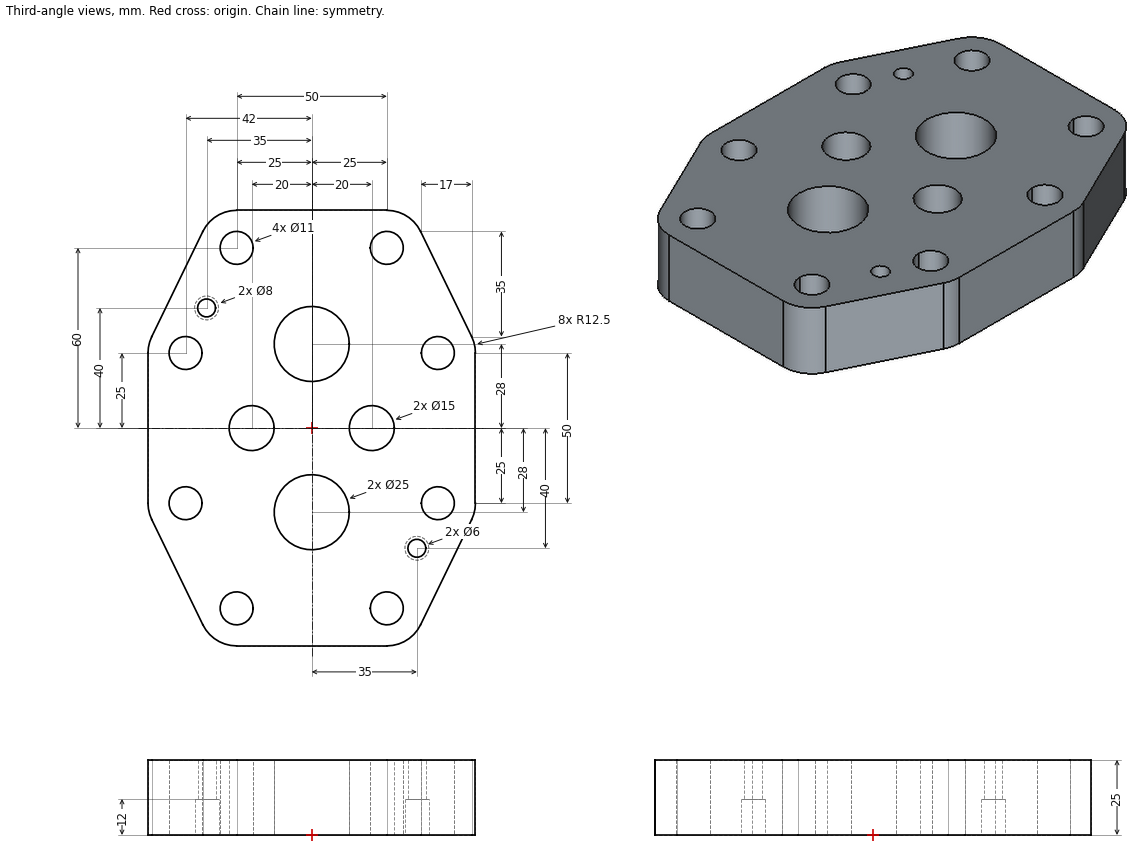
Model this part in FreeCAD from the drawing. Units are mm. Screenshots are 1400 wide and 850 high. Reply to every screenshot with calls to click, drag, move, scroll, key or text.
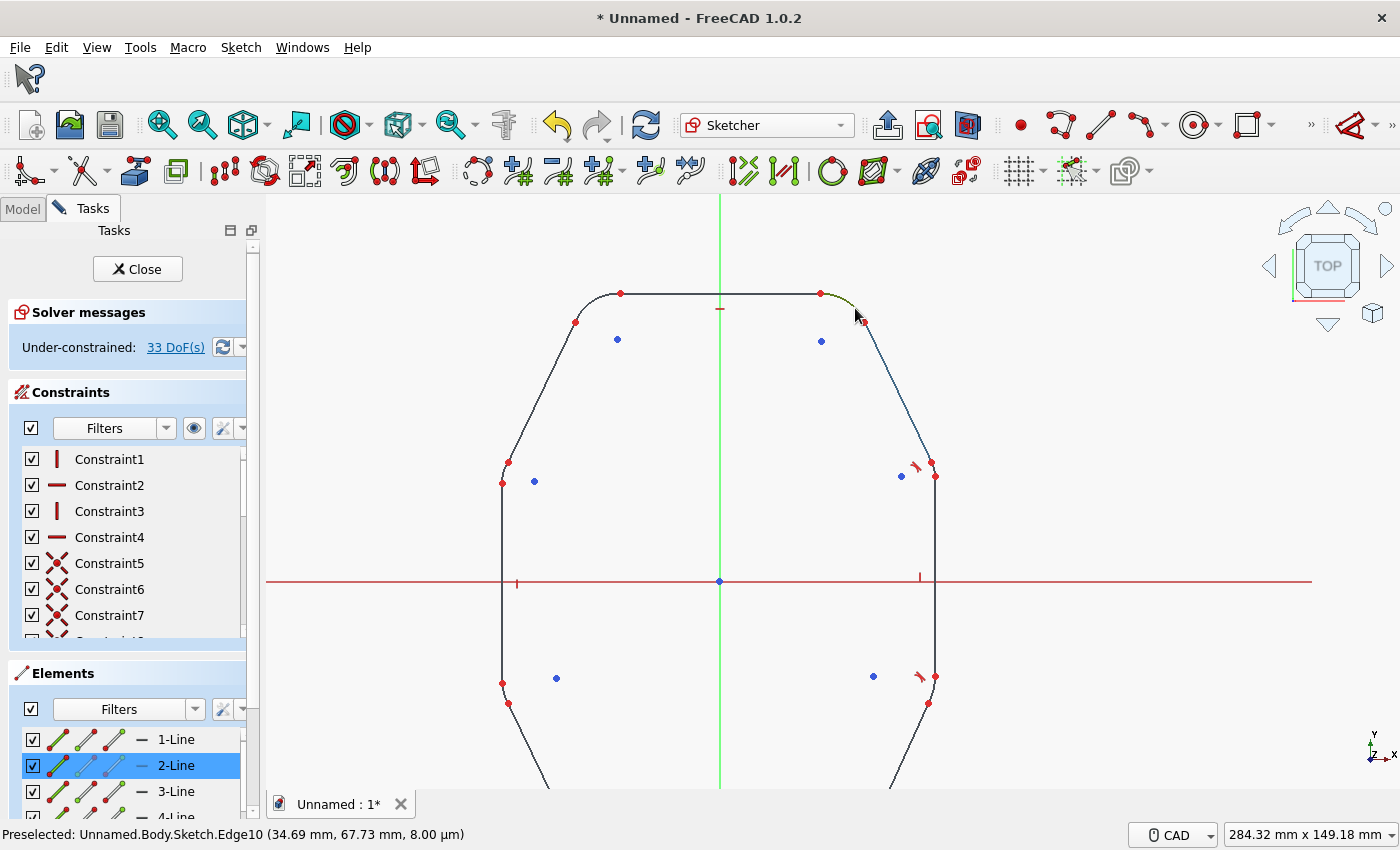
key(t)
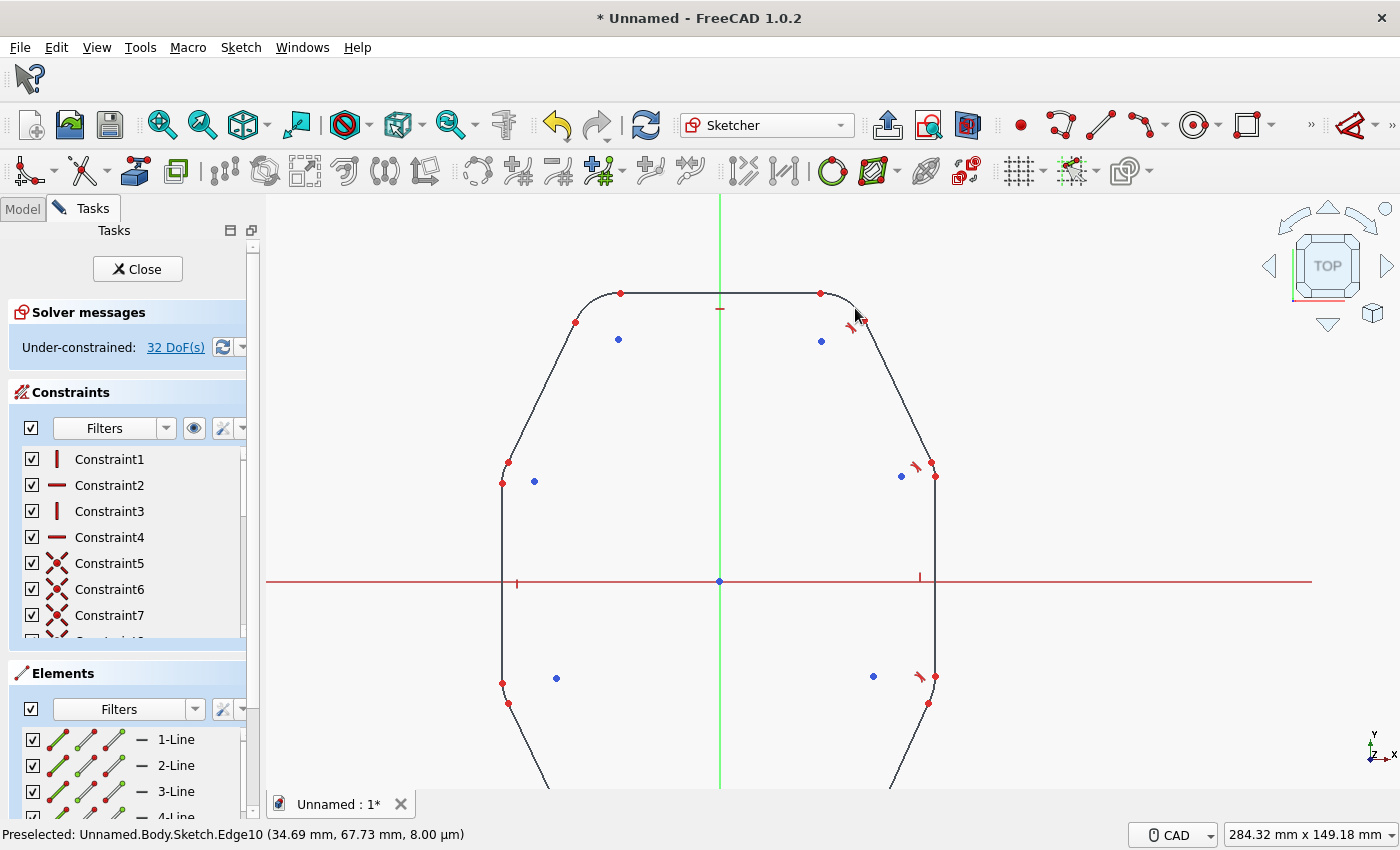
click(760, 293)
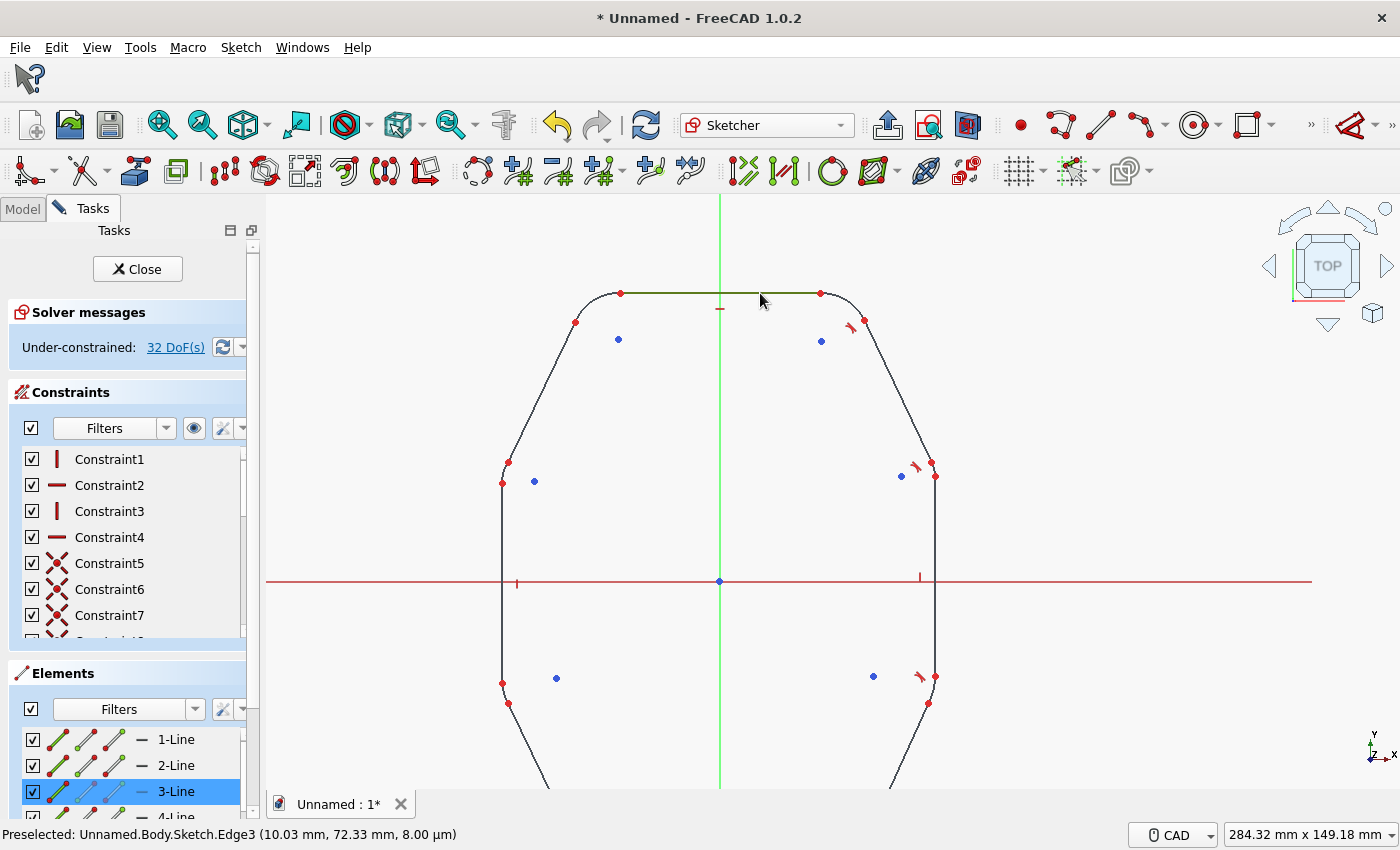
click(855, 307)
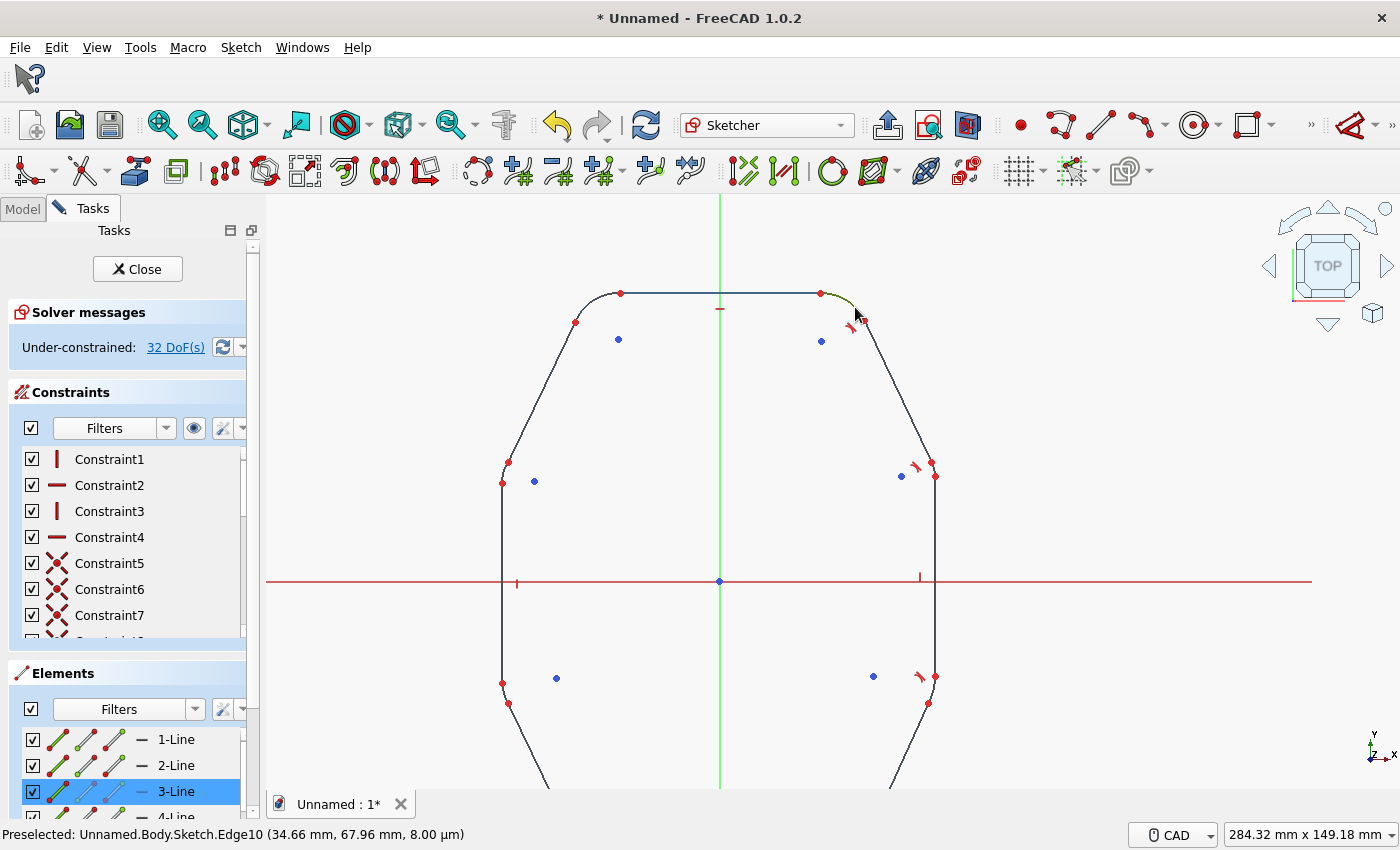
key(t)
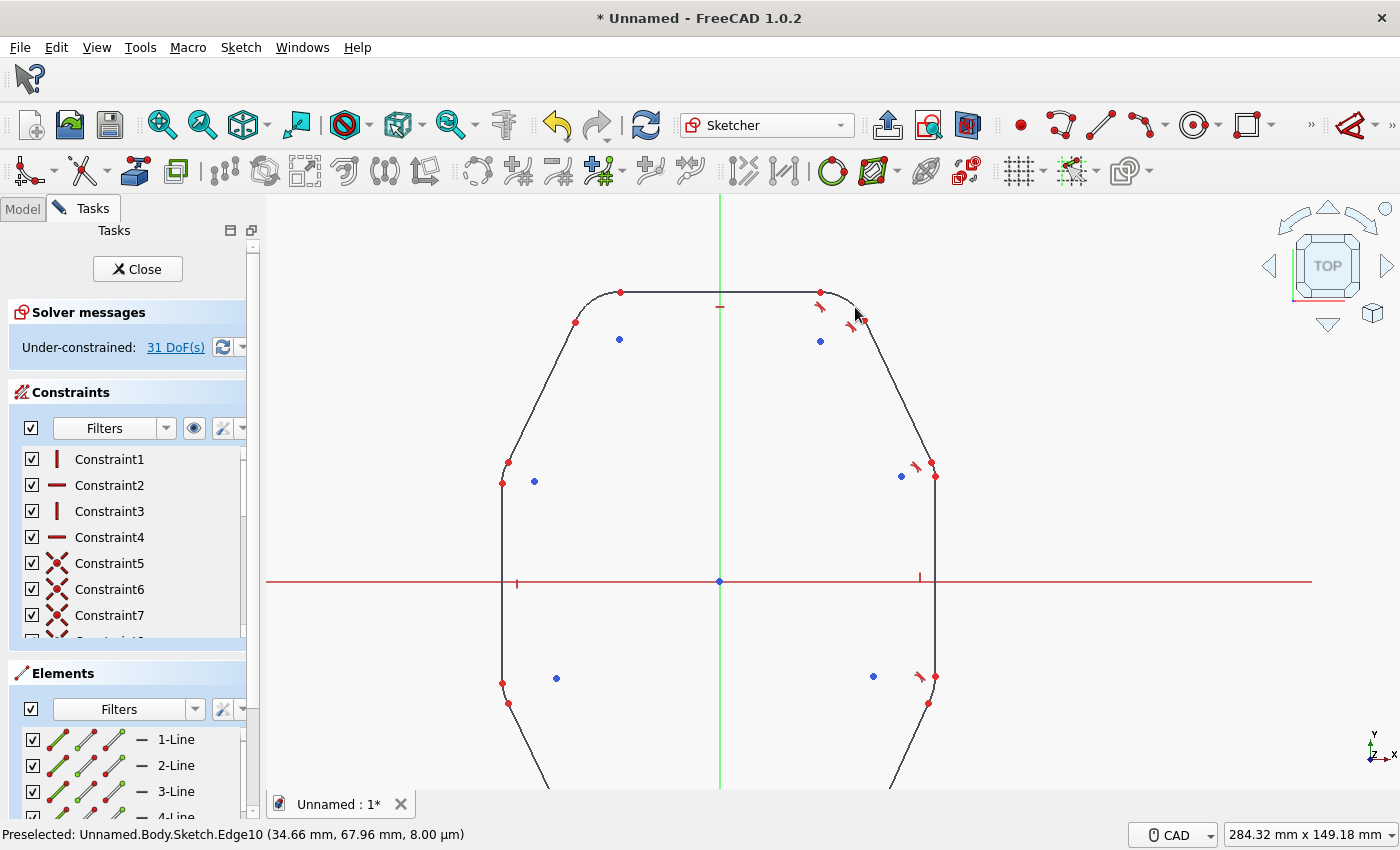
click(760, 292)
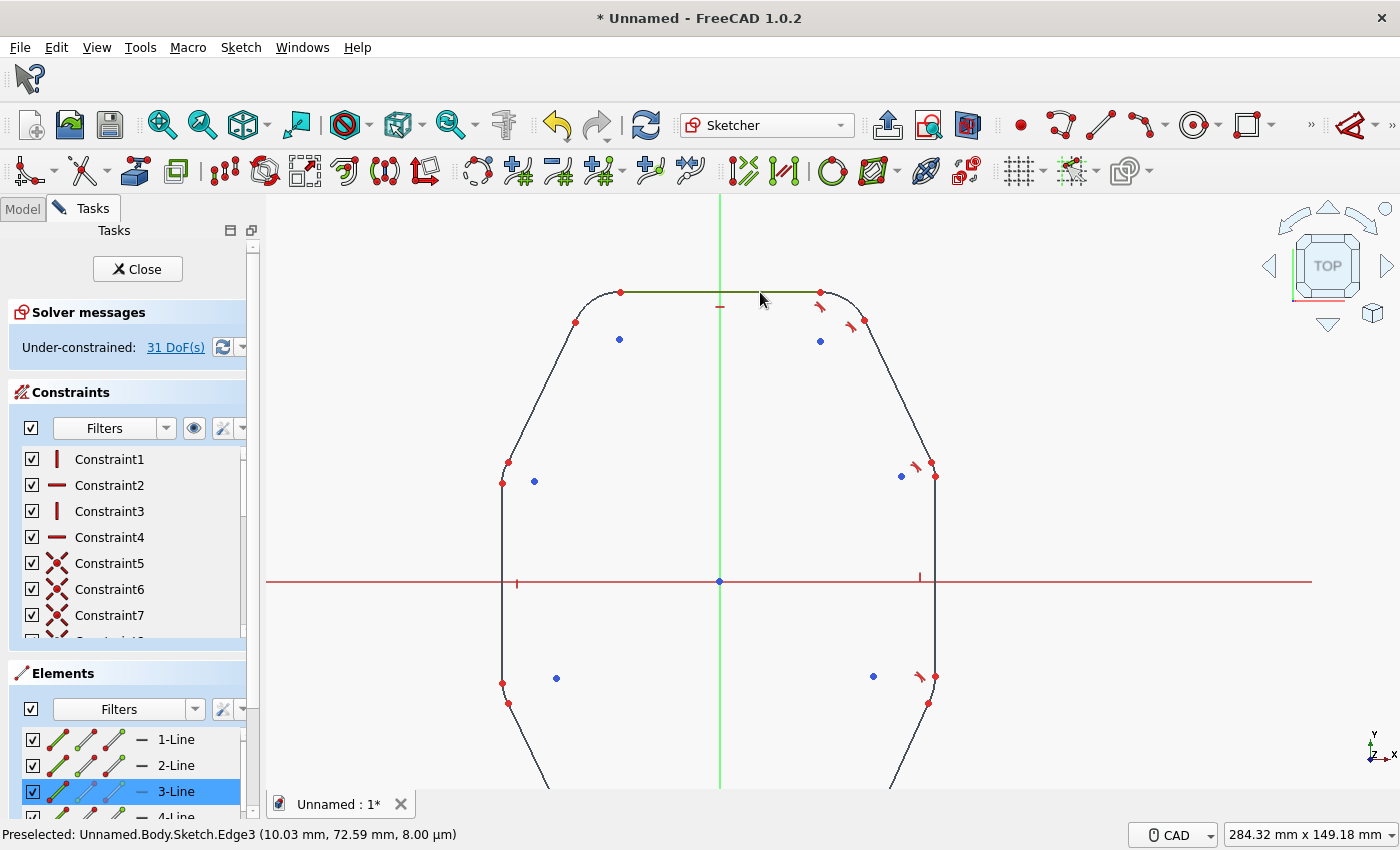
click(603, 295)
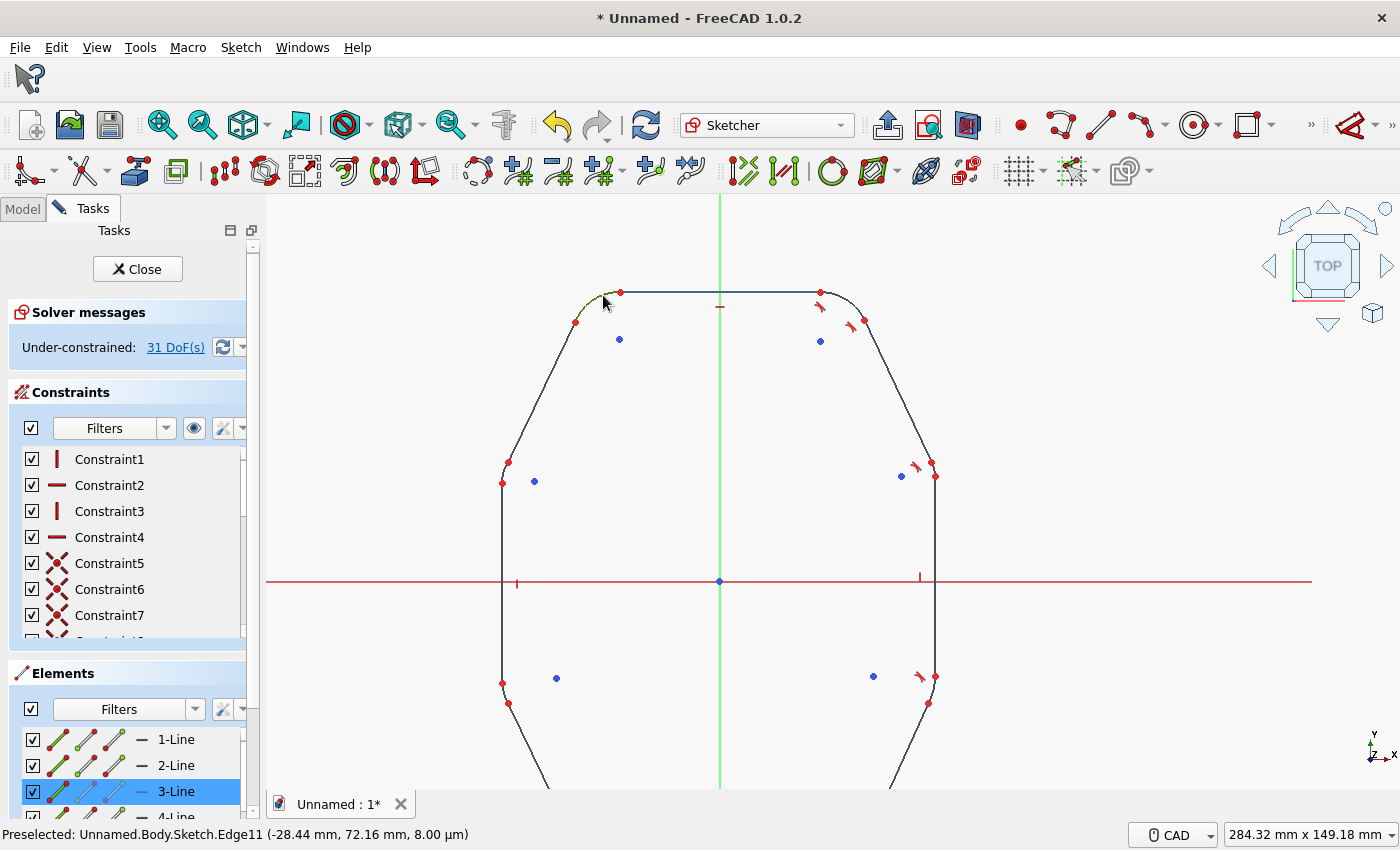
key(t)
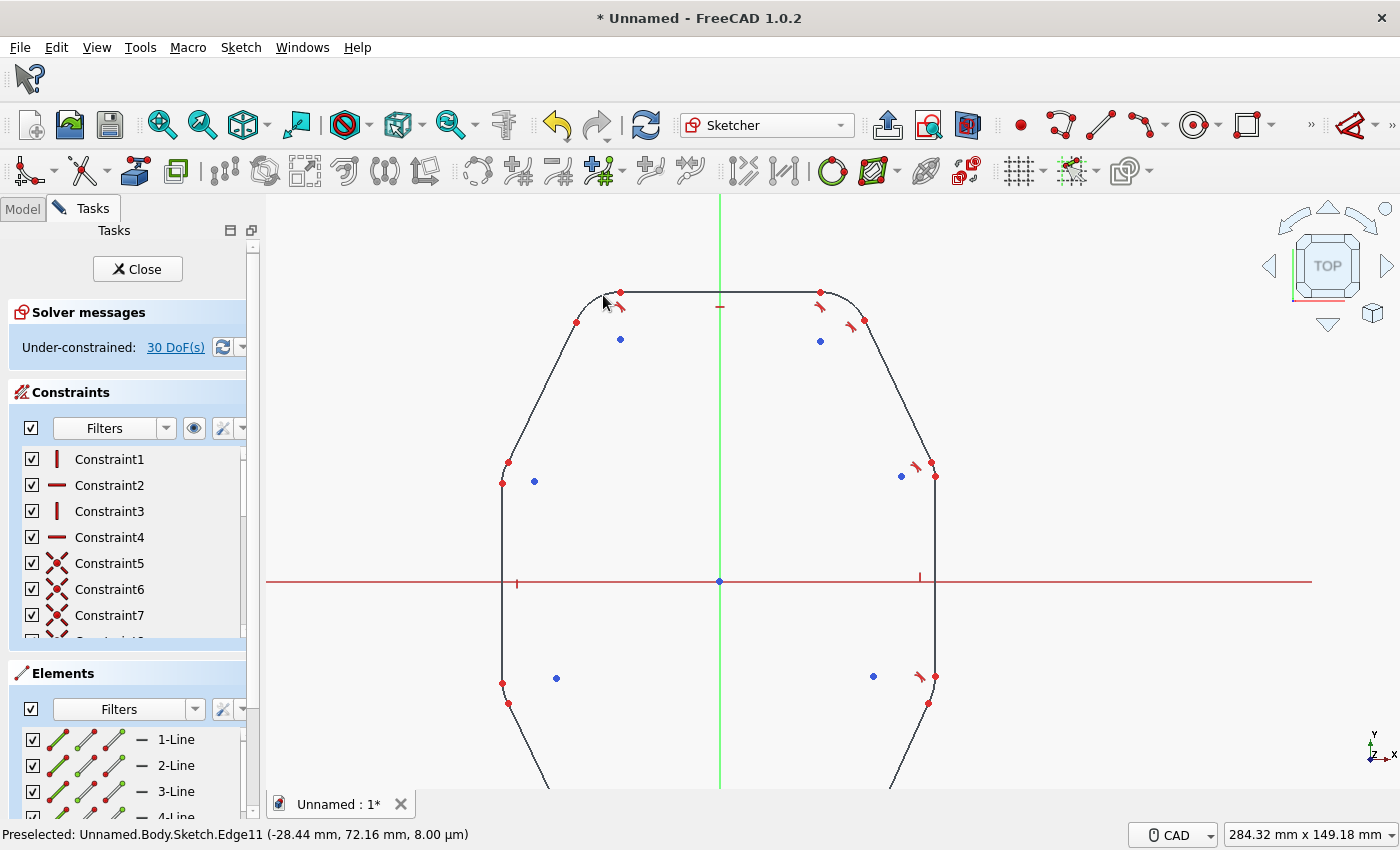
click(556, 364)